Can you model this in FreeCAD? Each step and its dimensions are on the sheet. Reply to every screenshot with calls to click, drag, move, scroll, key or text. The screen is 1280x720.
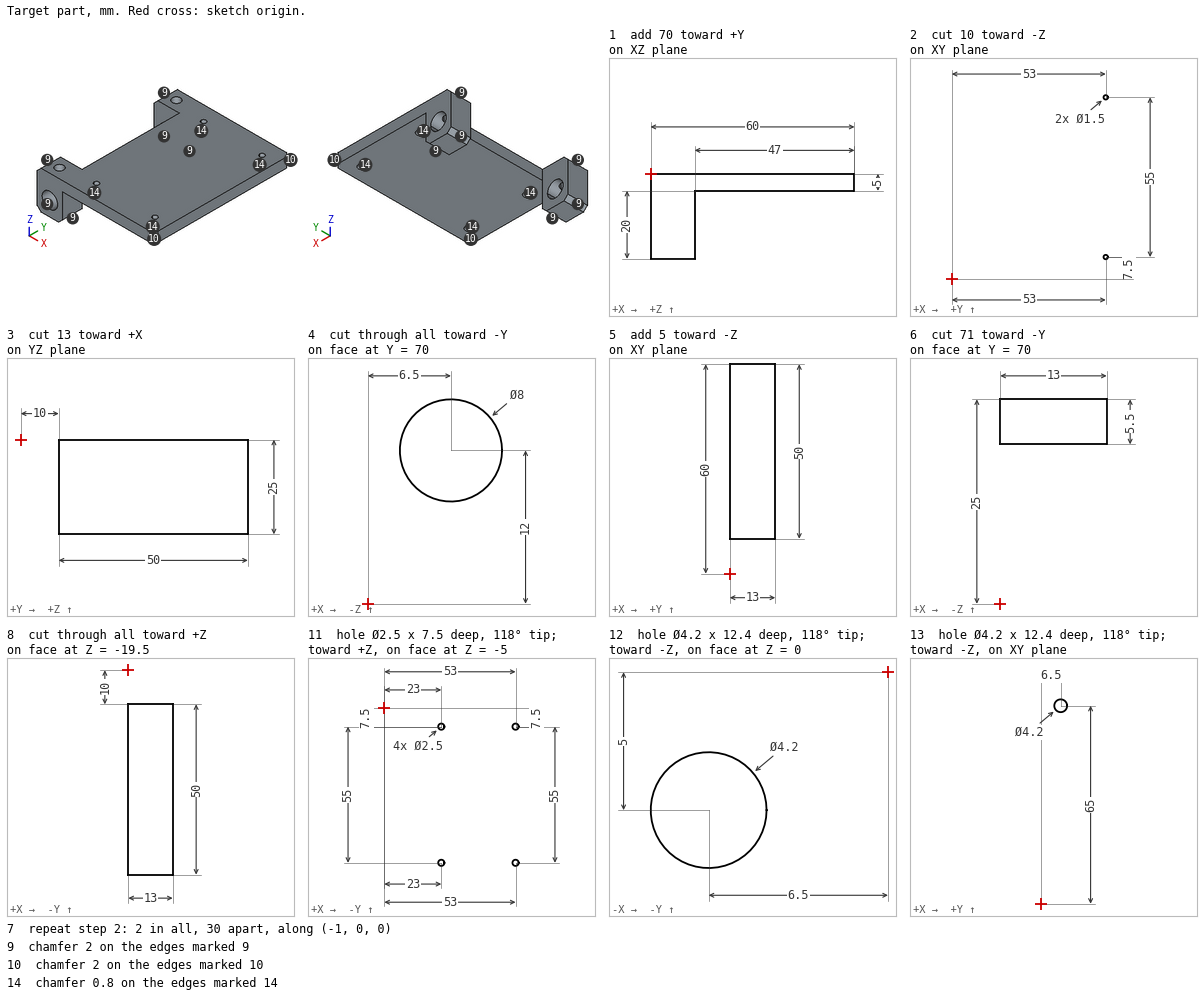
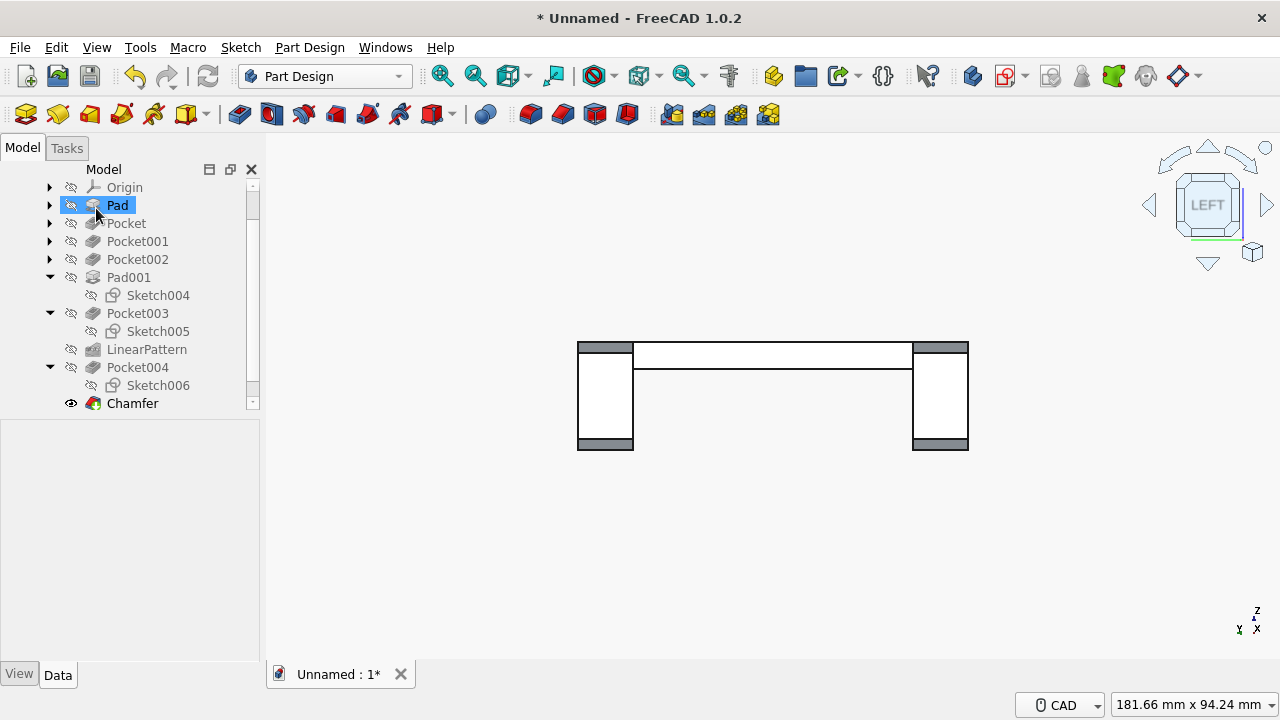
key(v)
key(f)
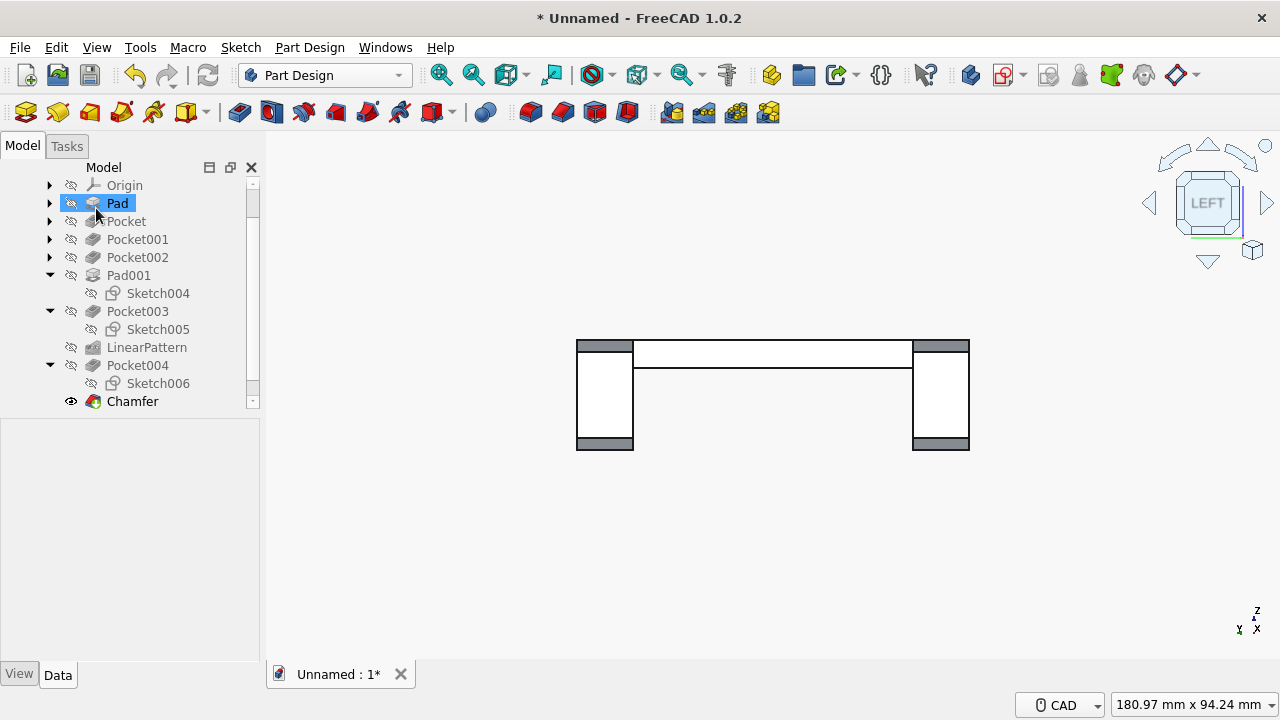
key(0)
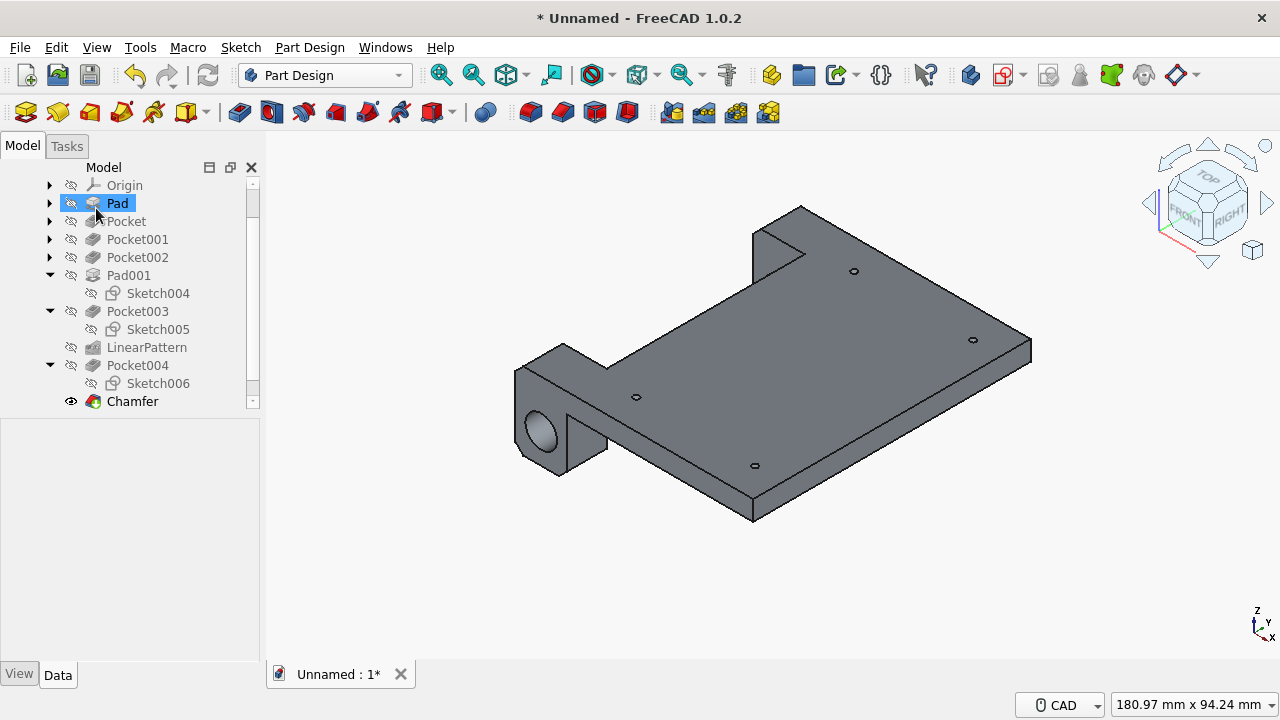
click(753, 510)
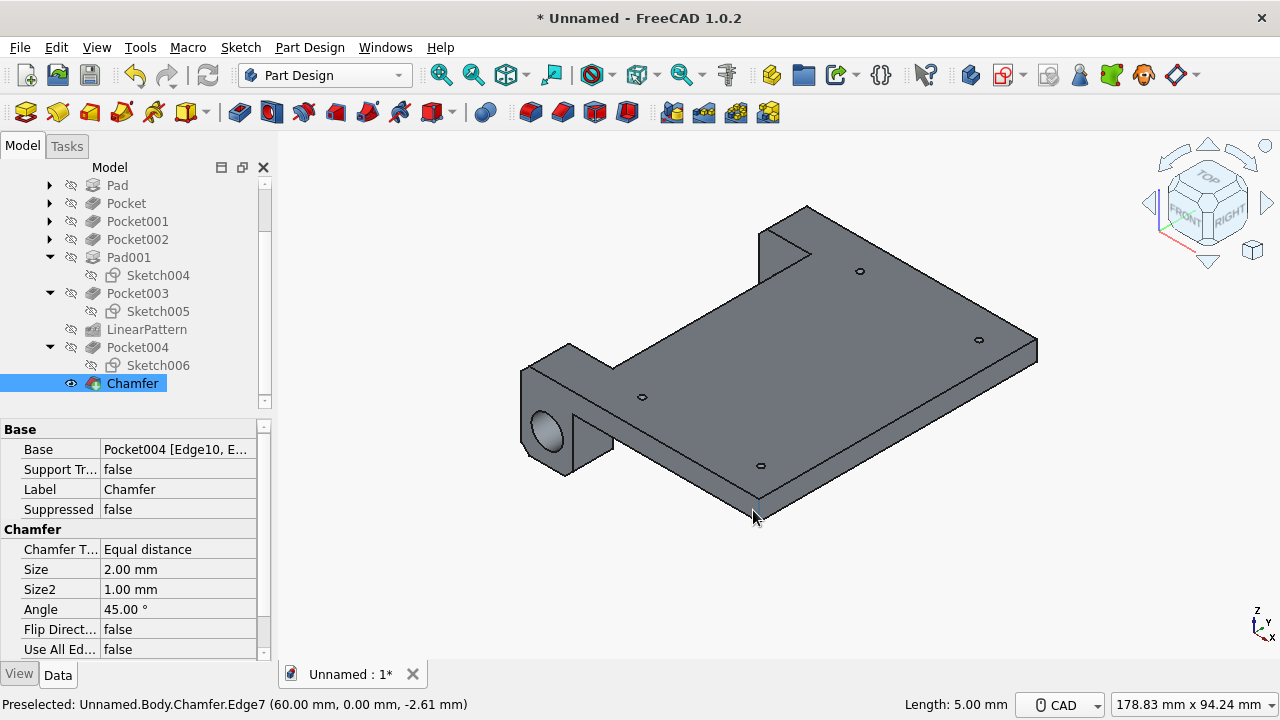
key(2)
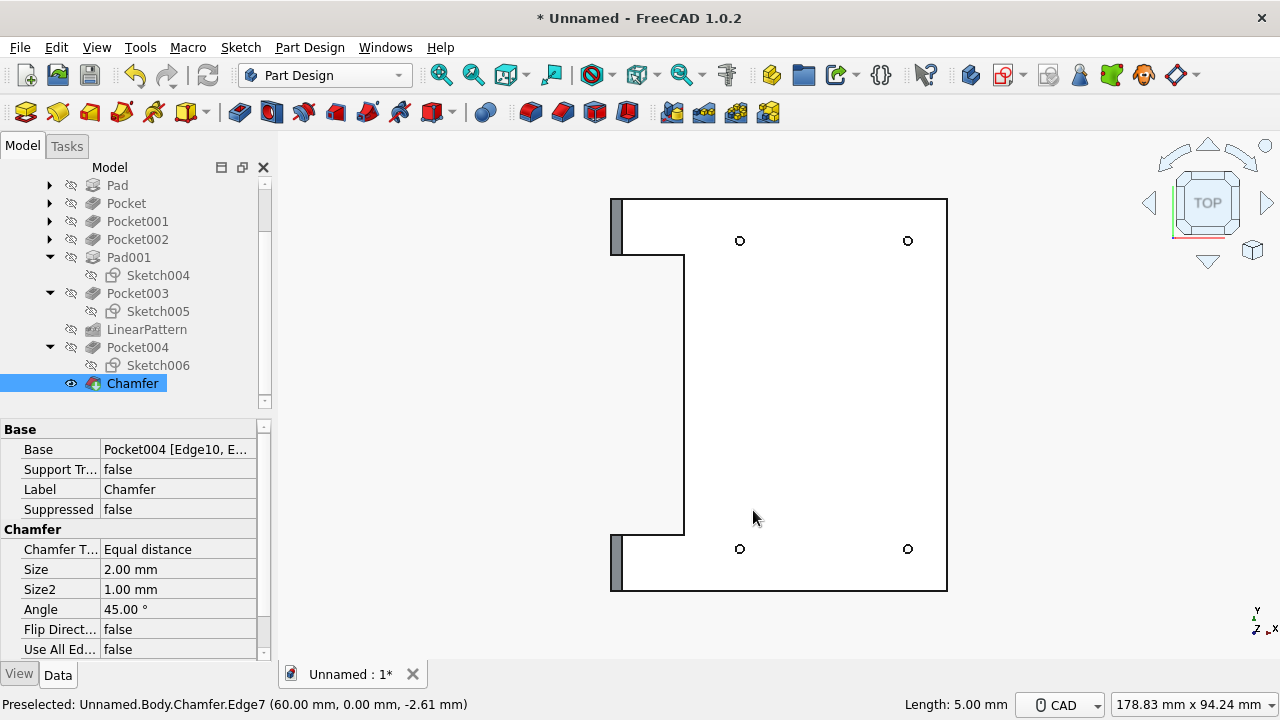
key(1)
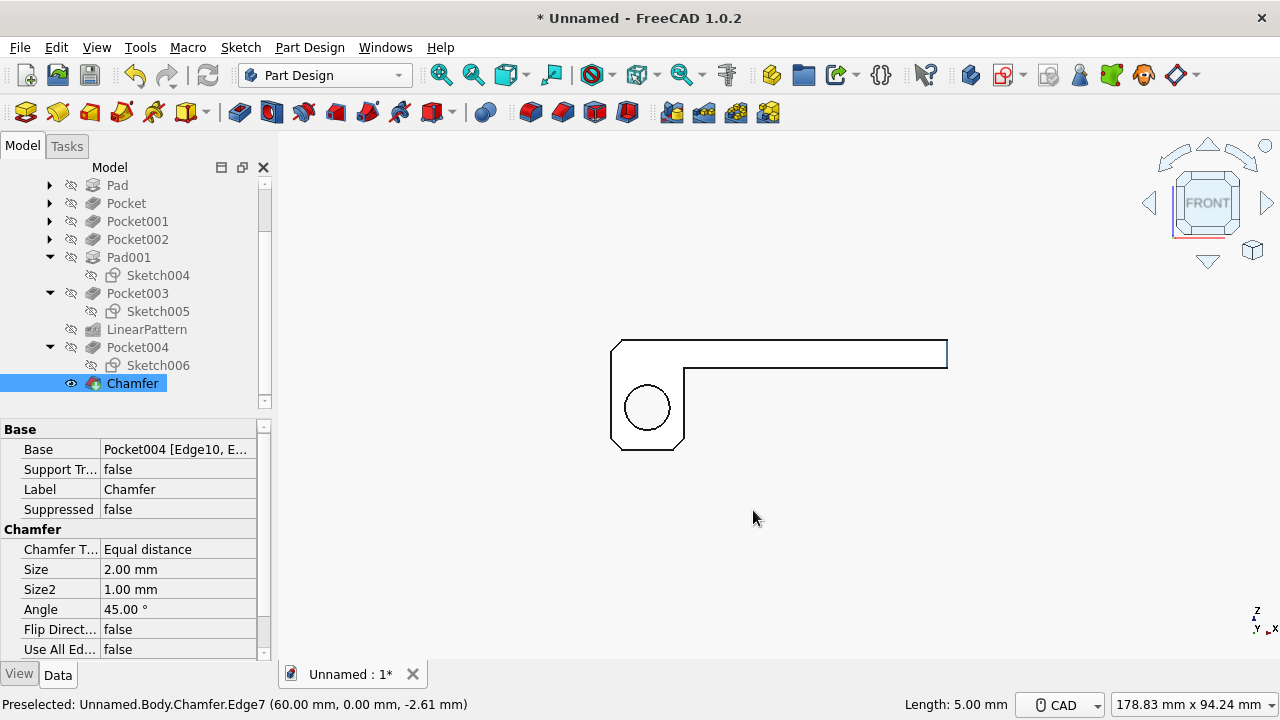
key(v)
key(f)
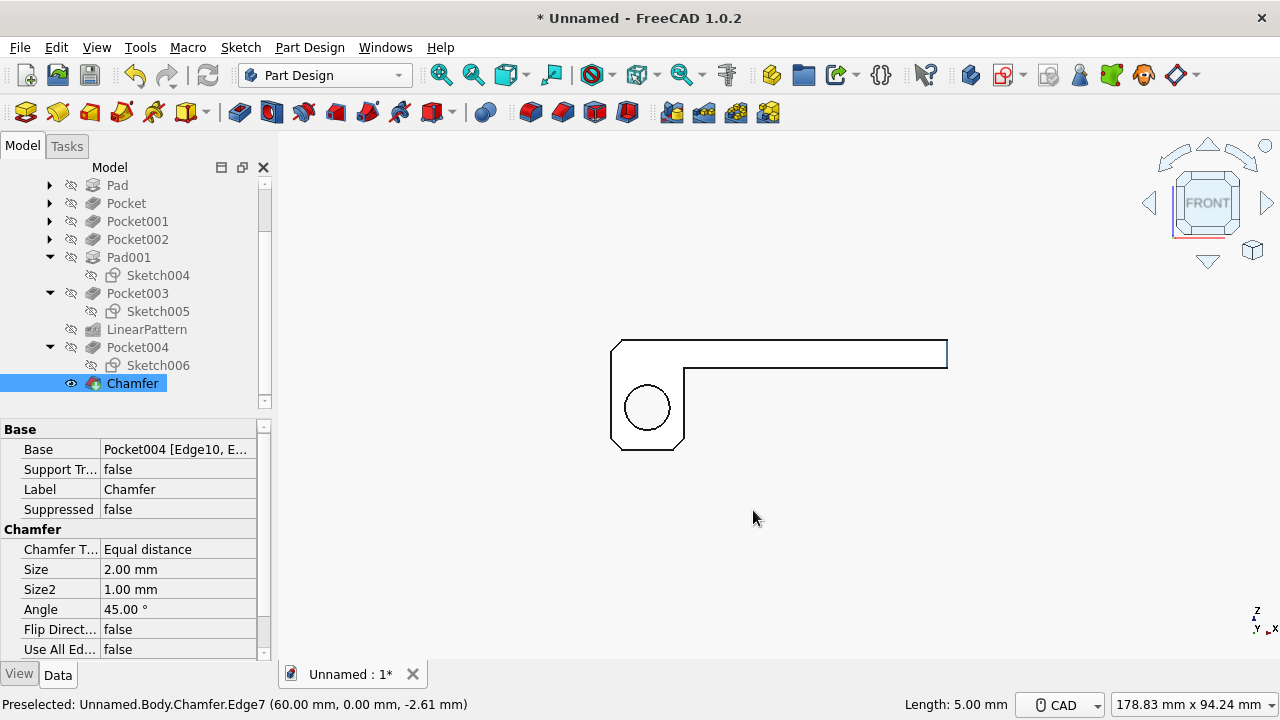
key(3)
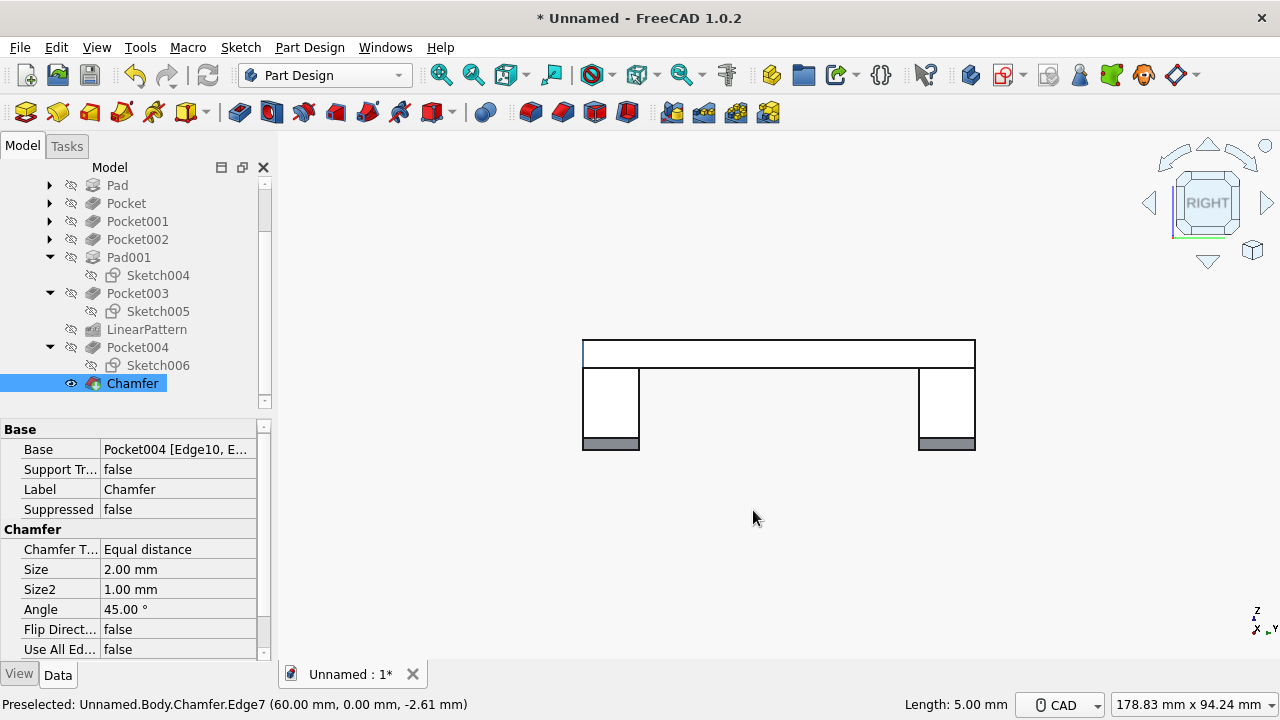
click(442, 76)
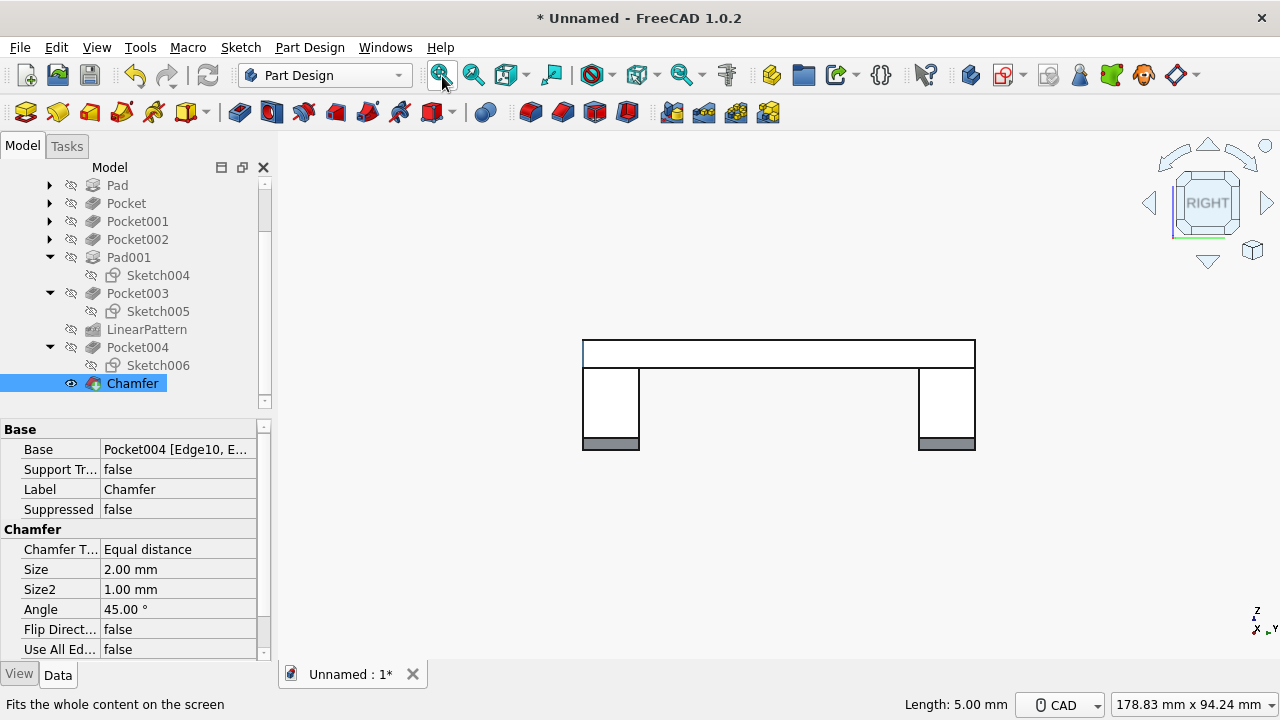
click(975, 353, ctrl)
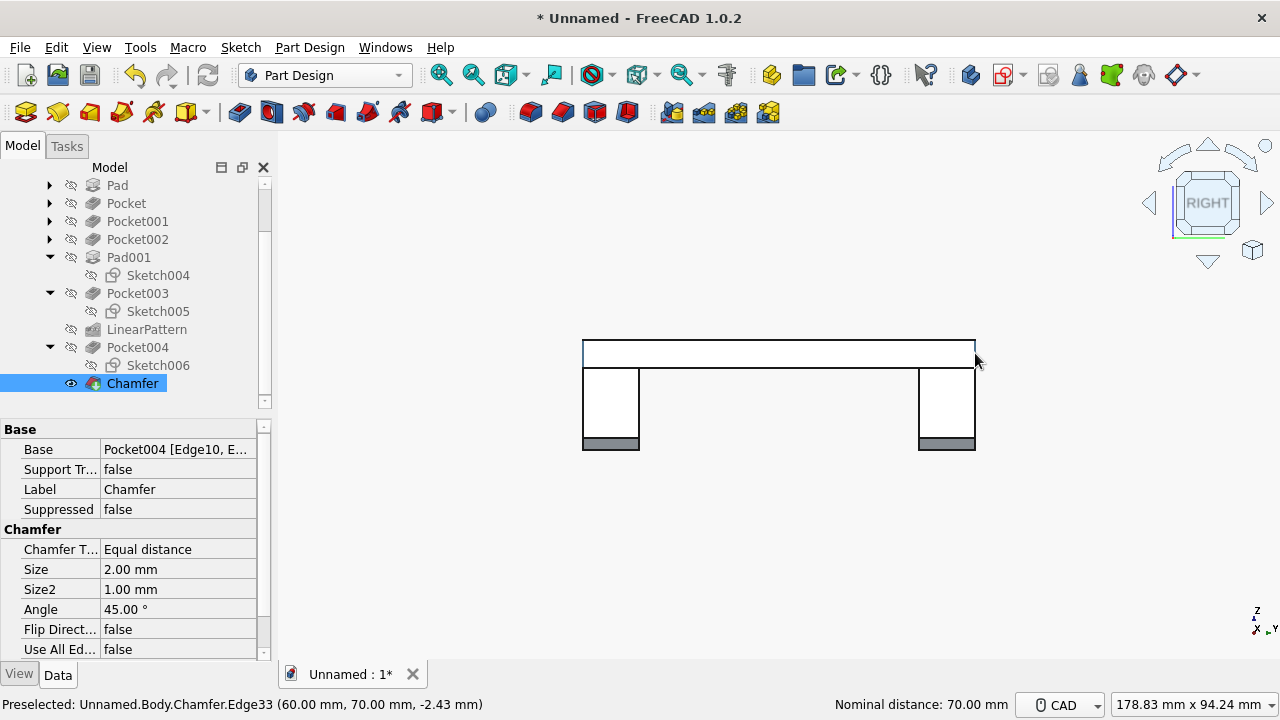
click(564, 112)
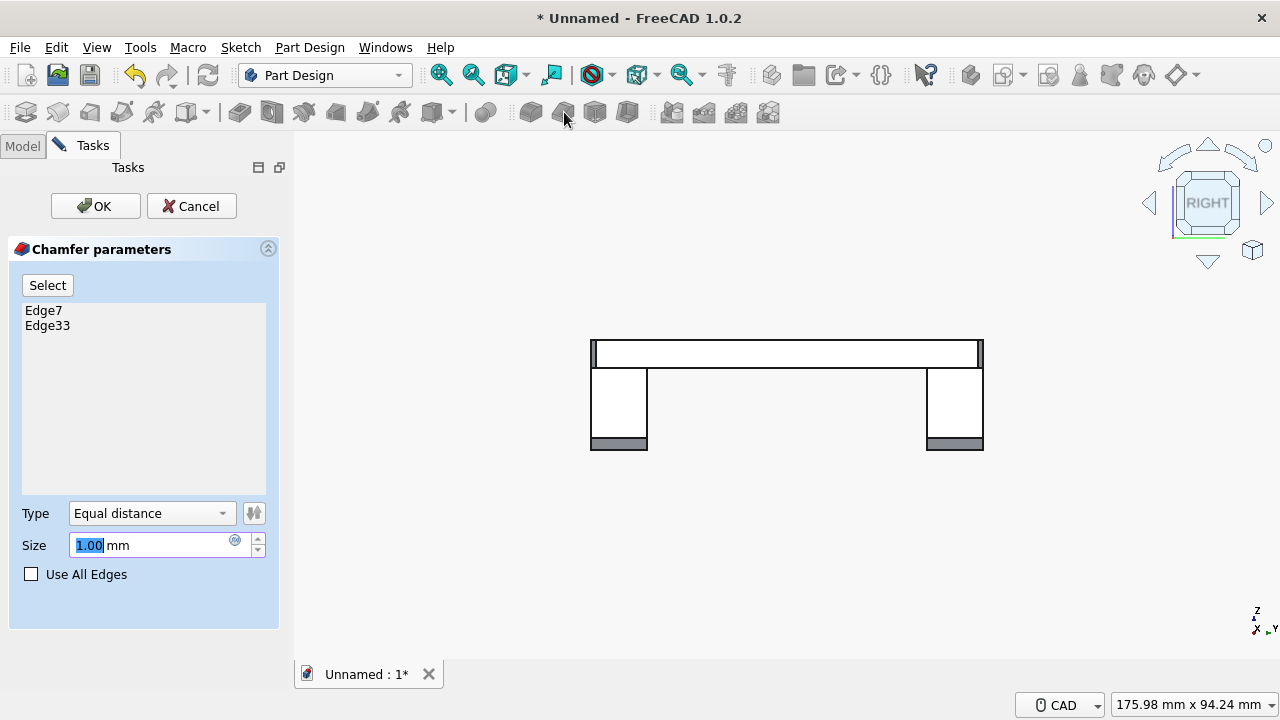
text(2)
key(Tab)